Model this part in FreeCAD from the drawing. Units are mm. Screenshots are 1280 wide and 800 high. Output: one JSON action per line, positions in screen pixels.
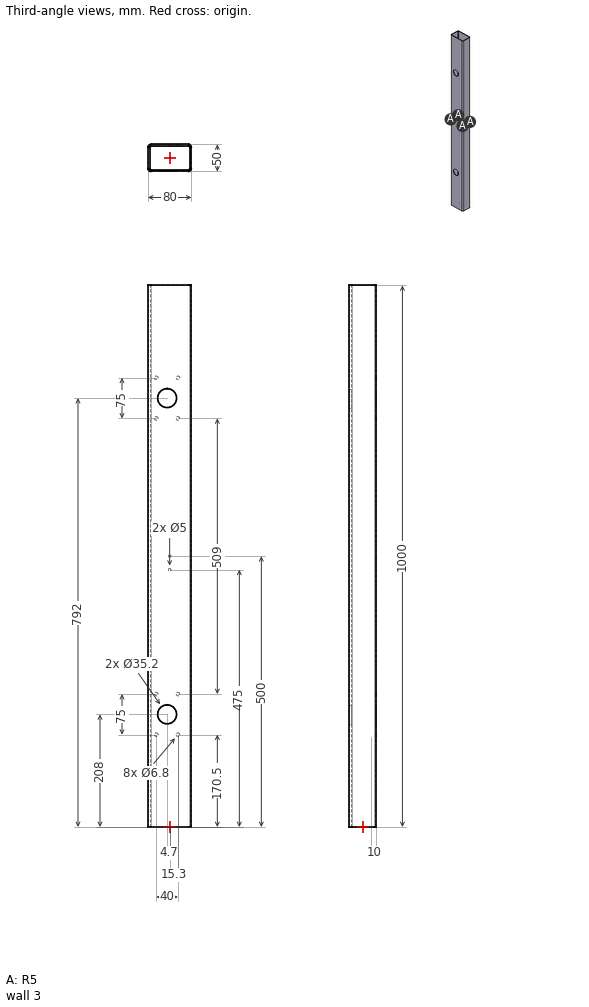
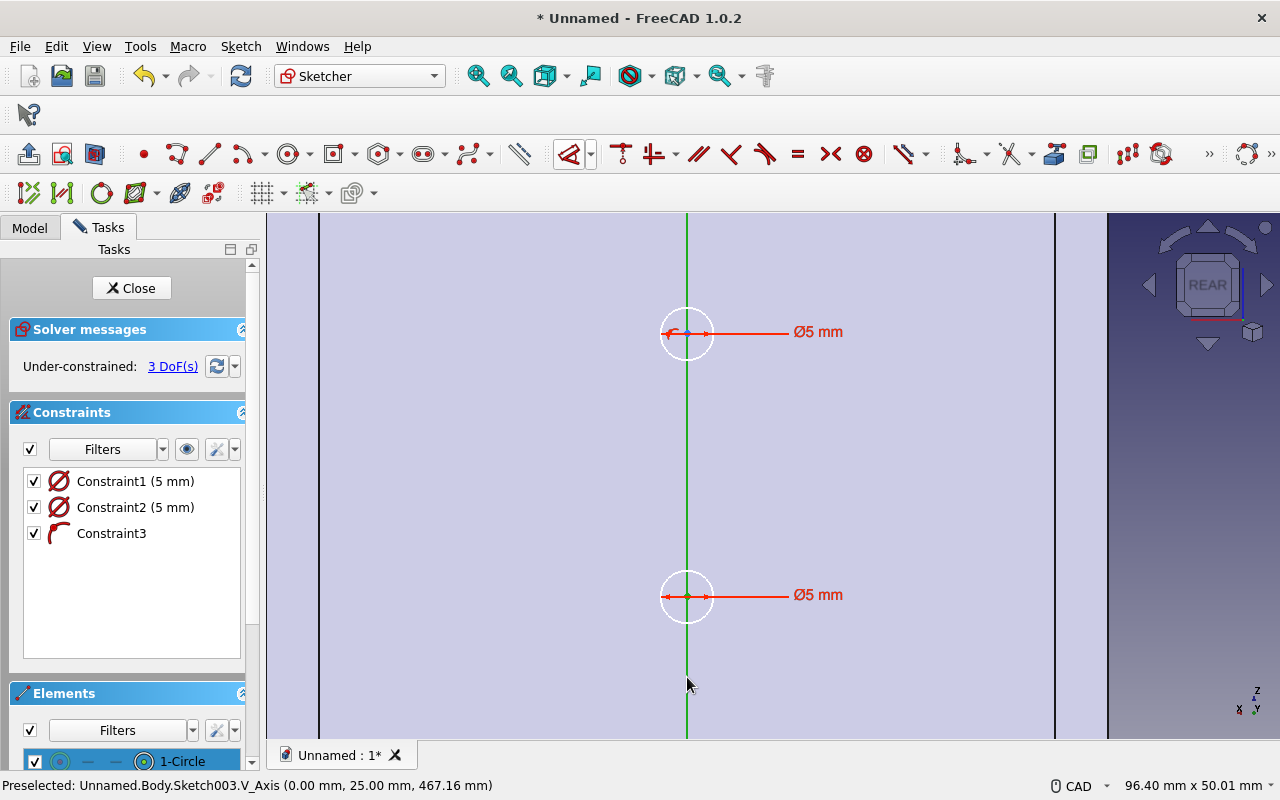
{"action": "left_click", "coordinate": [621, 154]}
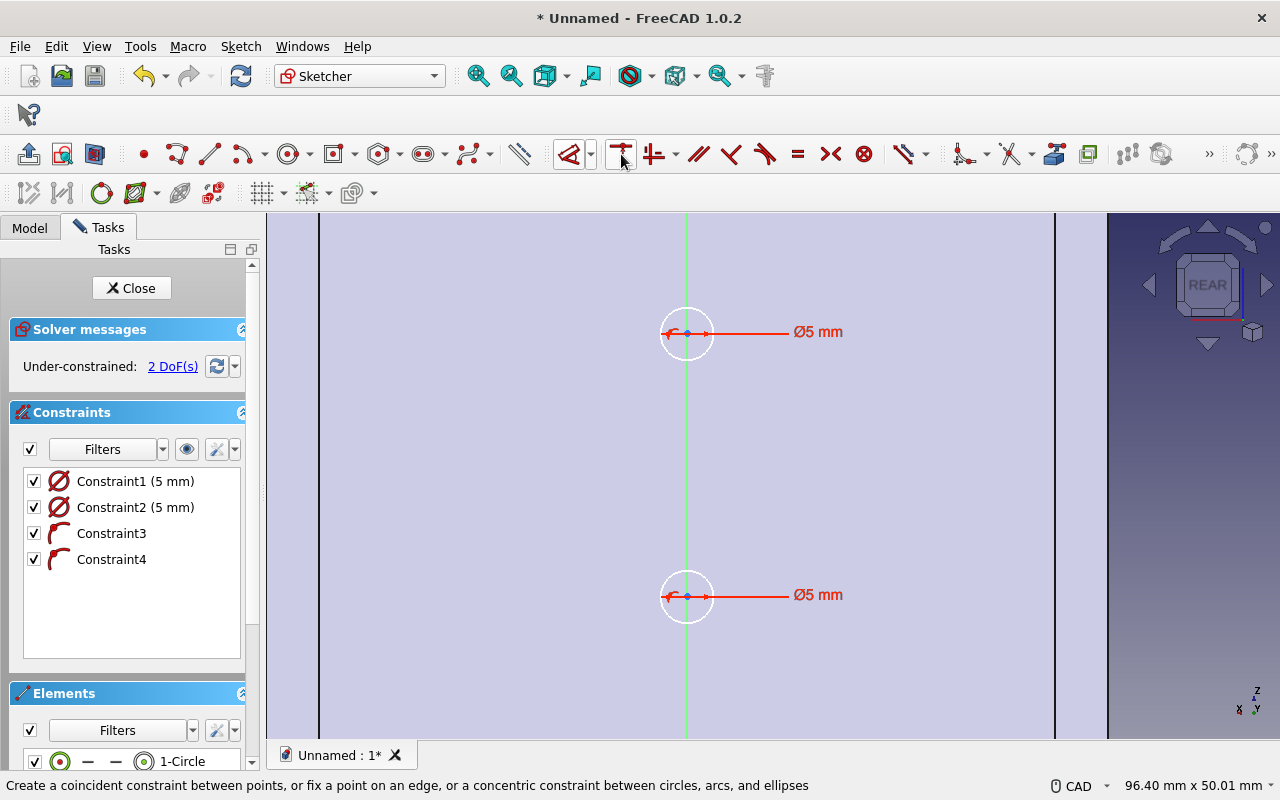
{"action": "left_click", "coordinate": [687, 597]}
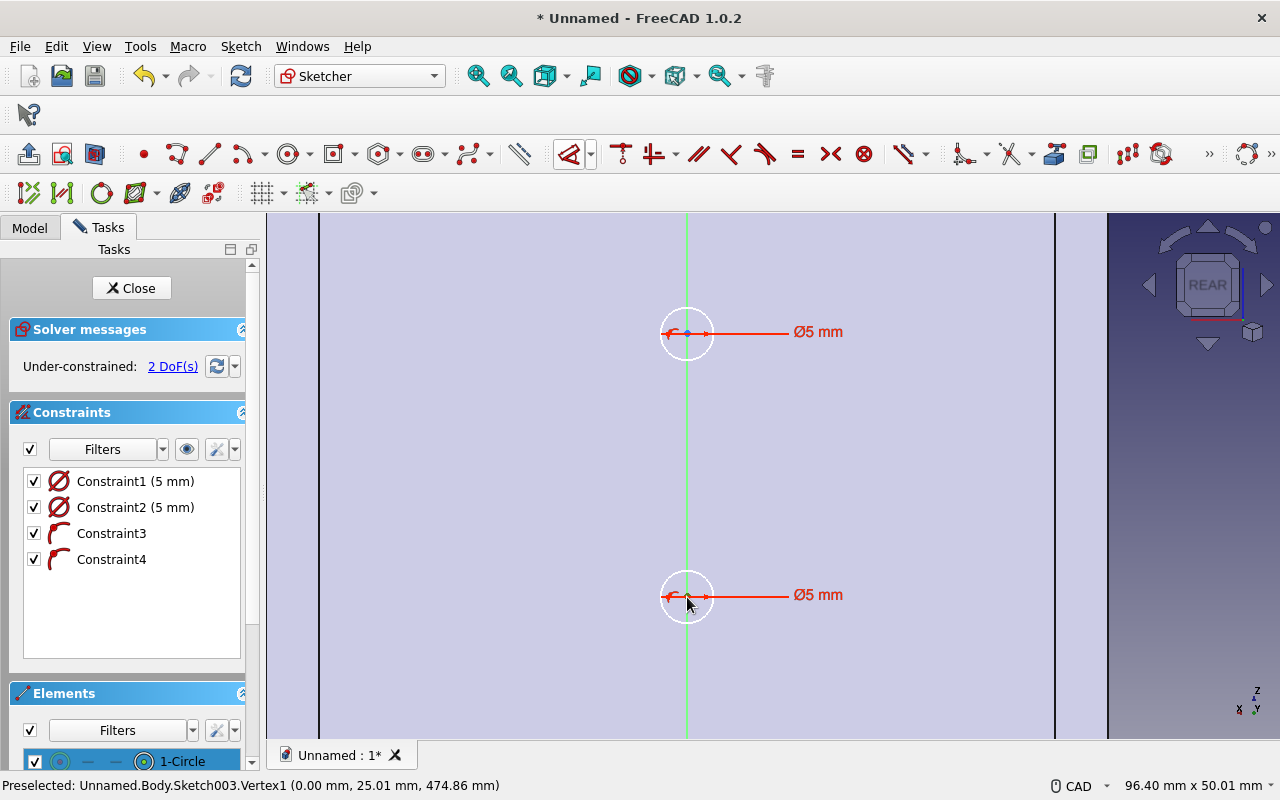
{"action": "left_click", "coordinate": [590, 154]}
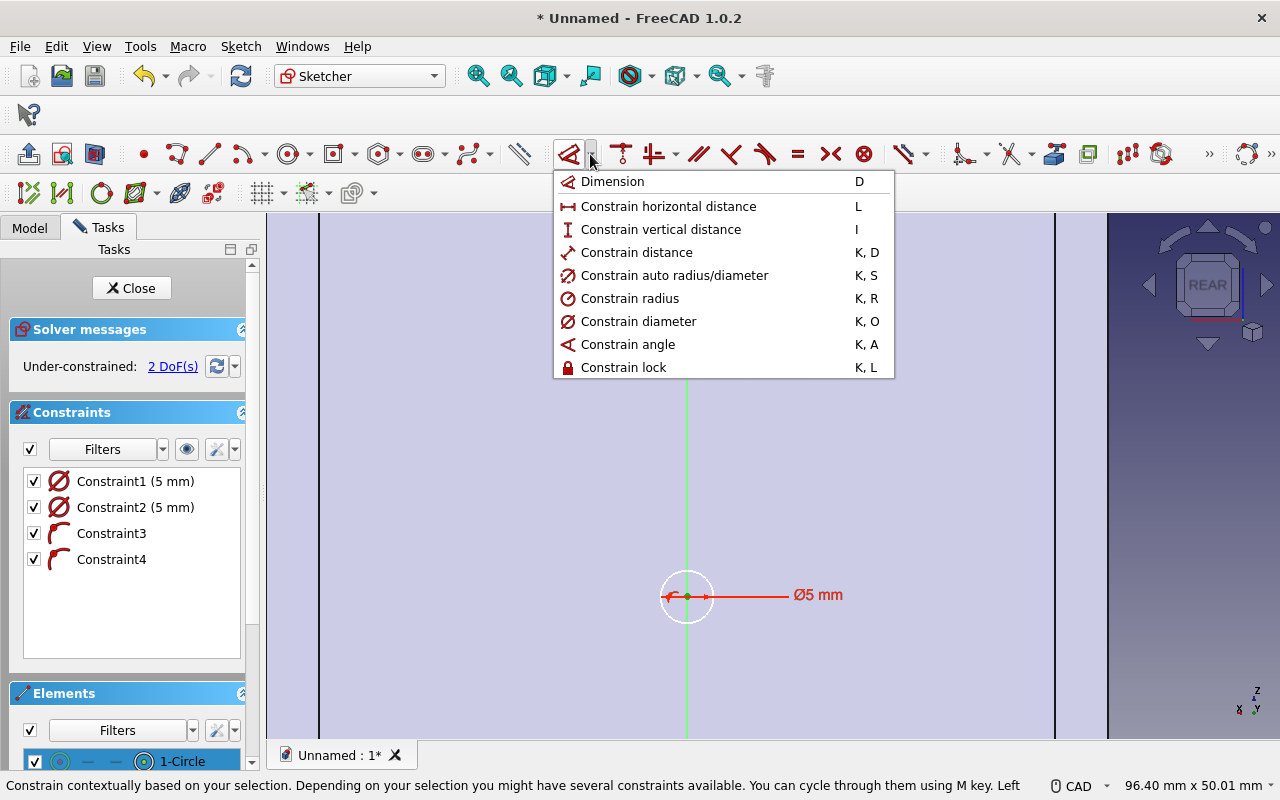
{"action": "left_click", "coordinate": [724, 230]}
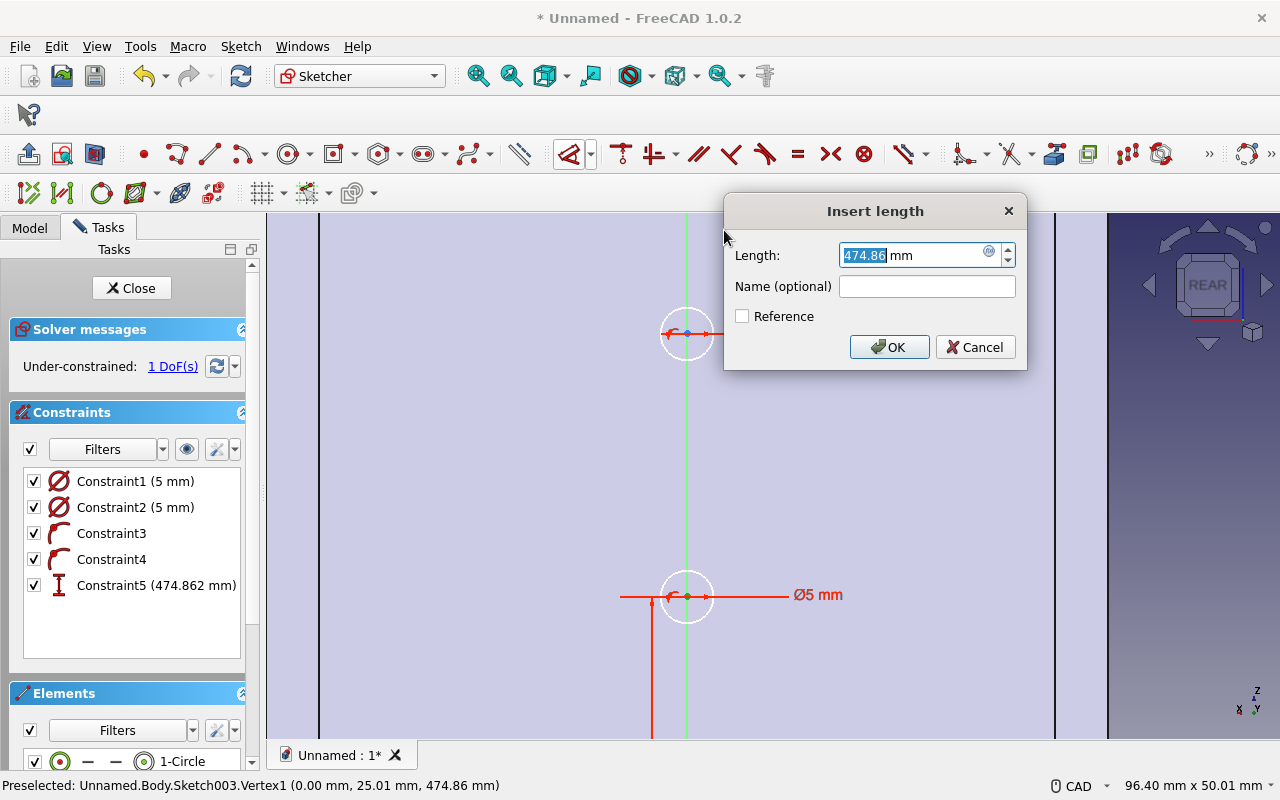
{"action": "type", "text": "475"}
{"action": "key", "text": "Return"}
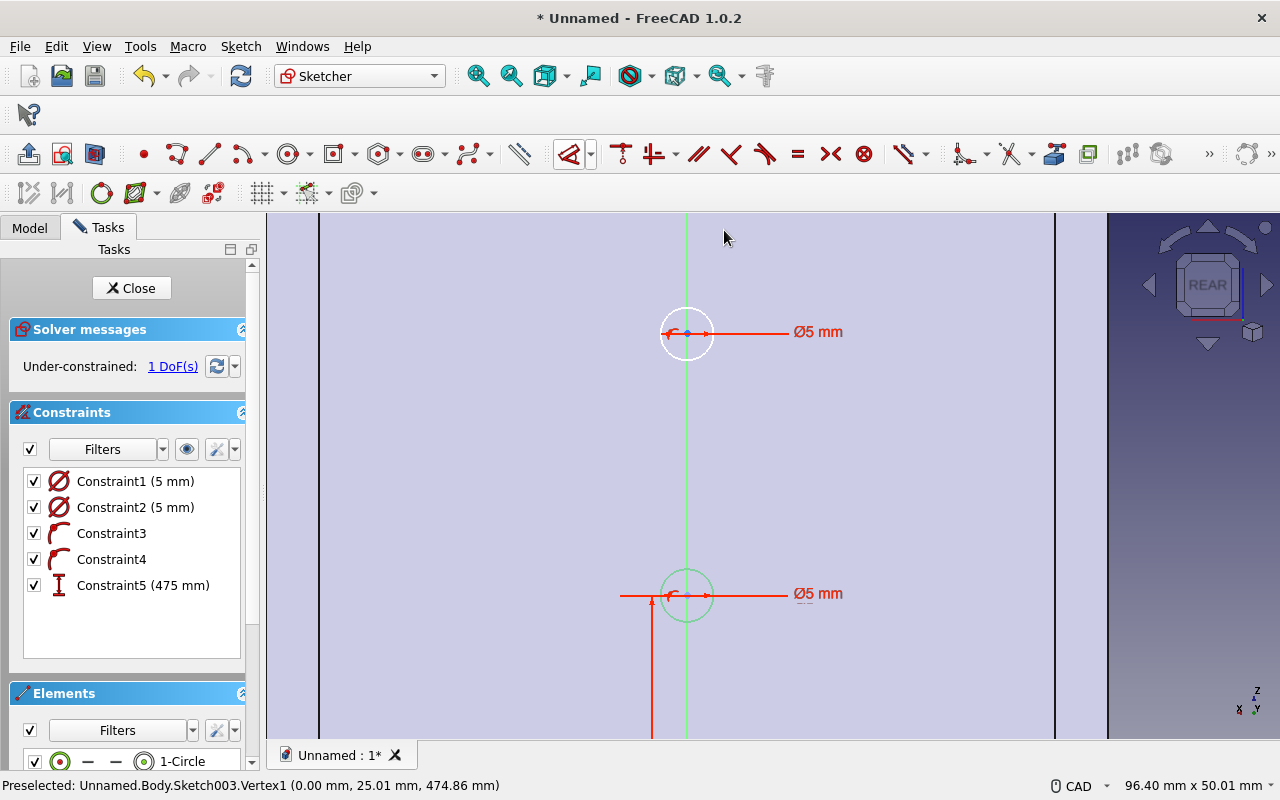
{"action": "left_click", "coordinate": [687, 334]}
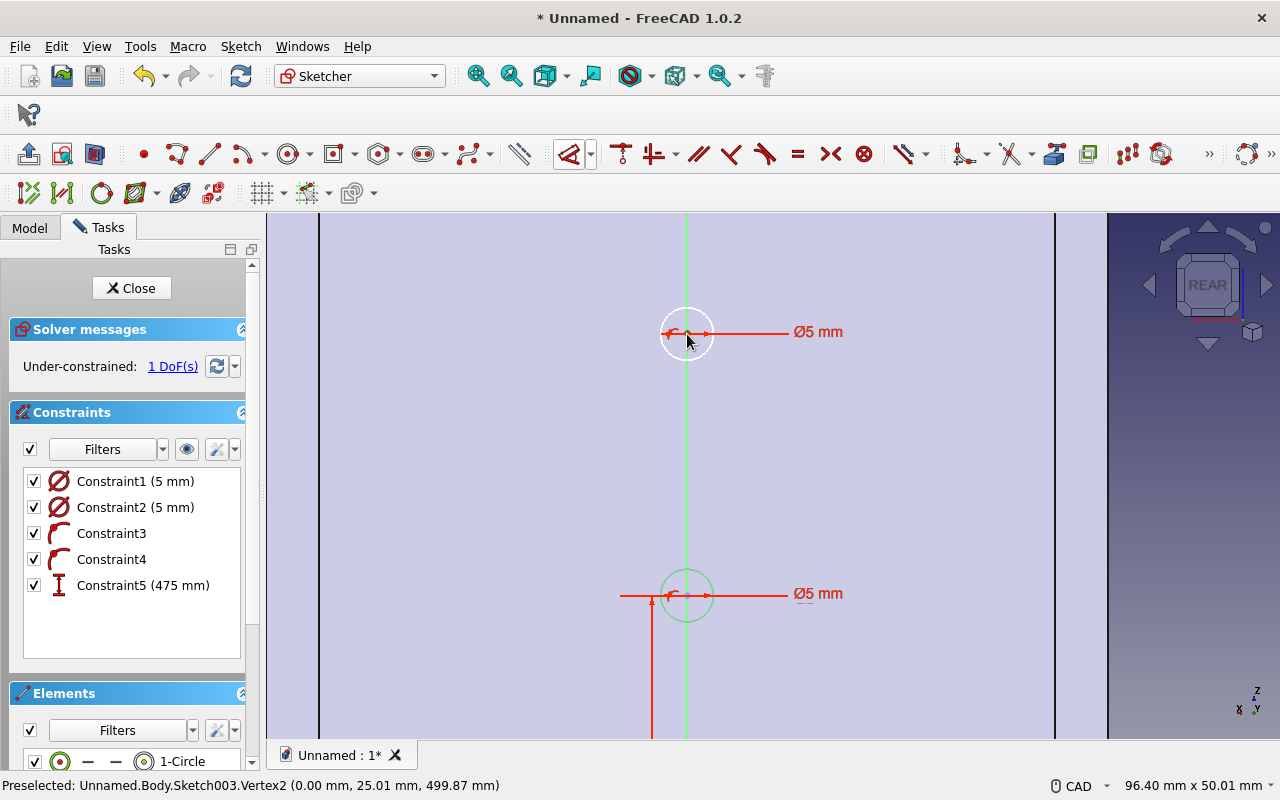
{"action": "left_click", "coordinate": [590, 154]}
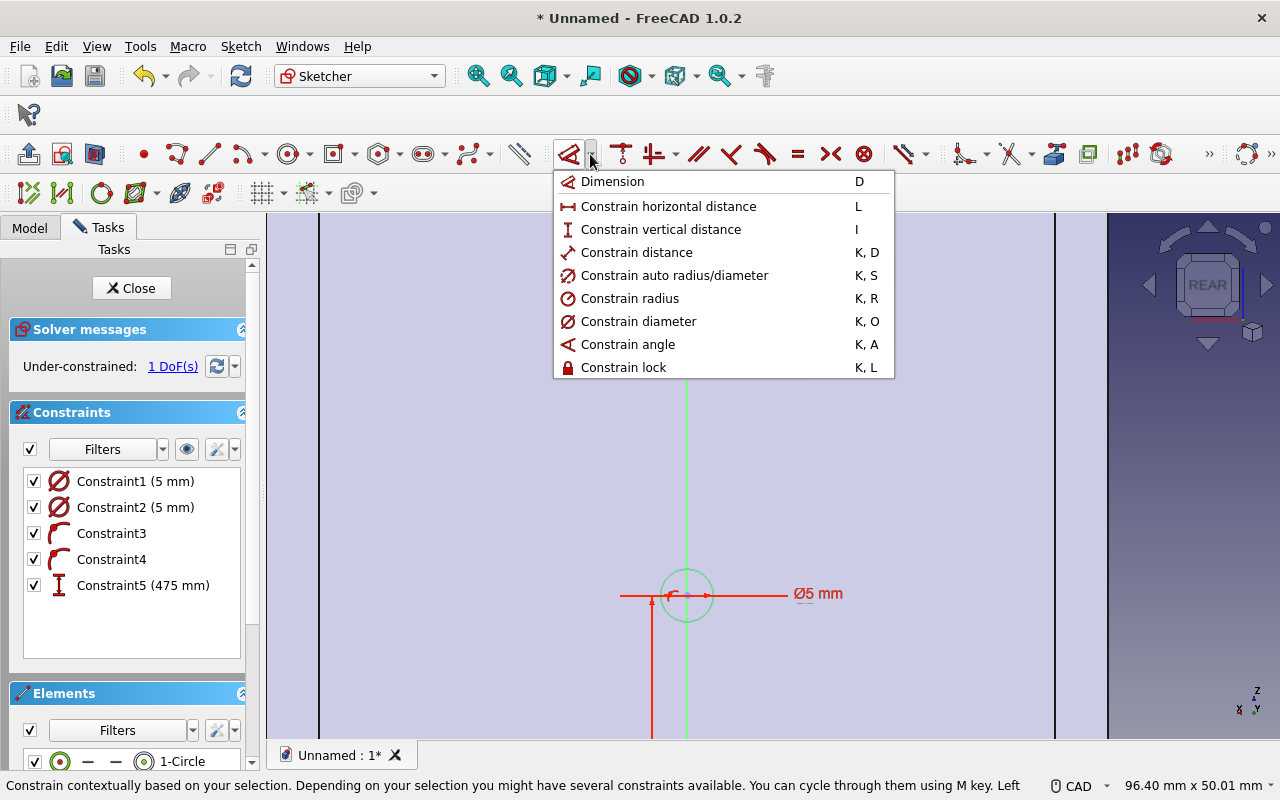
{"action": "left_click", "coordinate": [724, 230]}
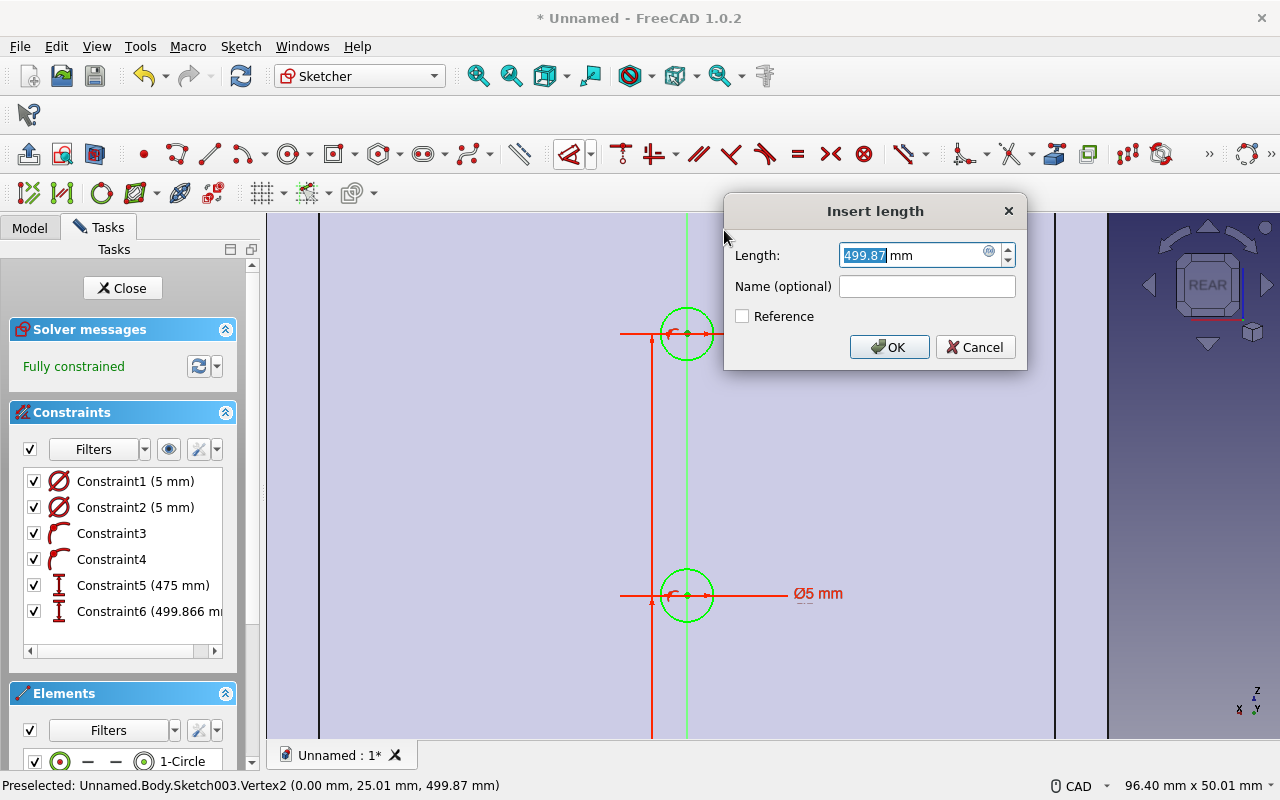
{"action": "type", "text": "500"}
{"action": "key", "text": "Return"}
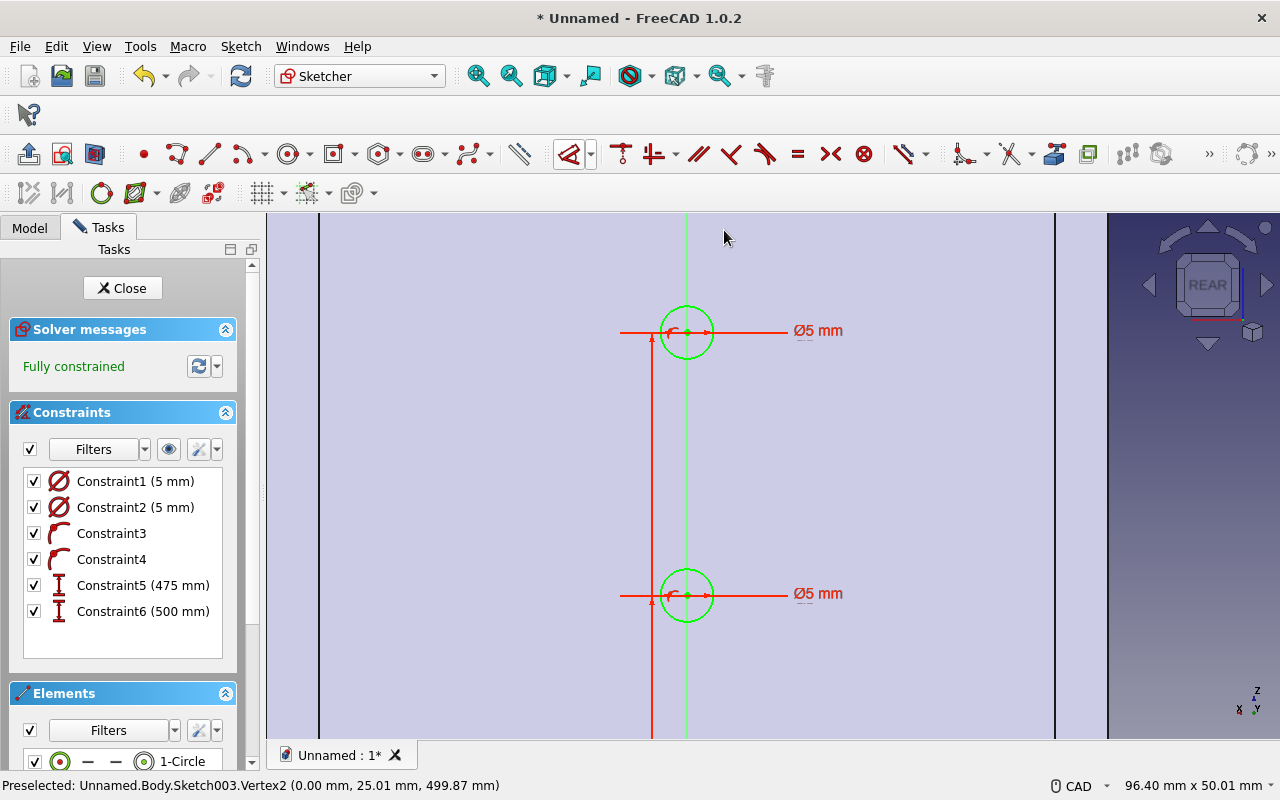
{"action": "left_click", "coordinate": [123, 288]}